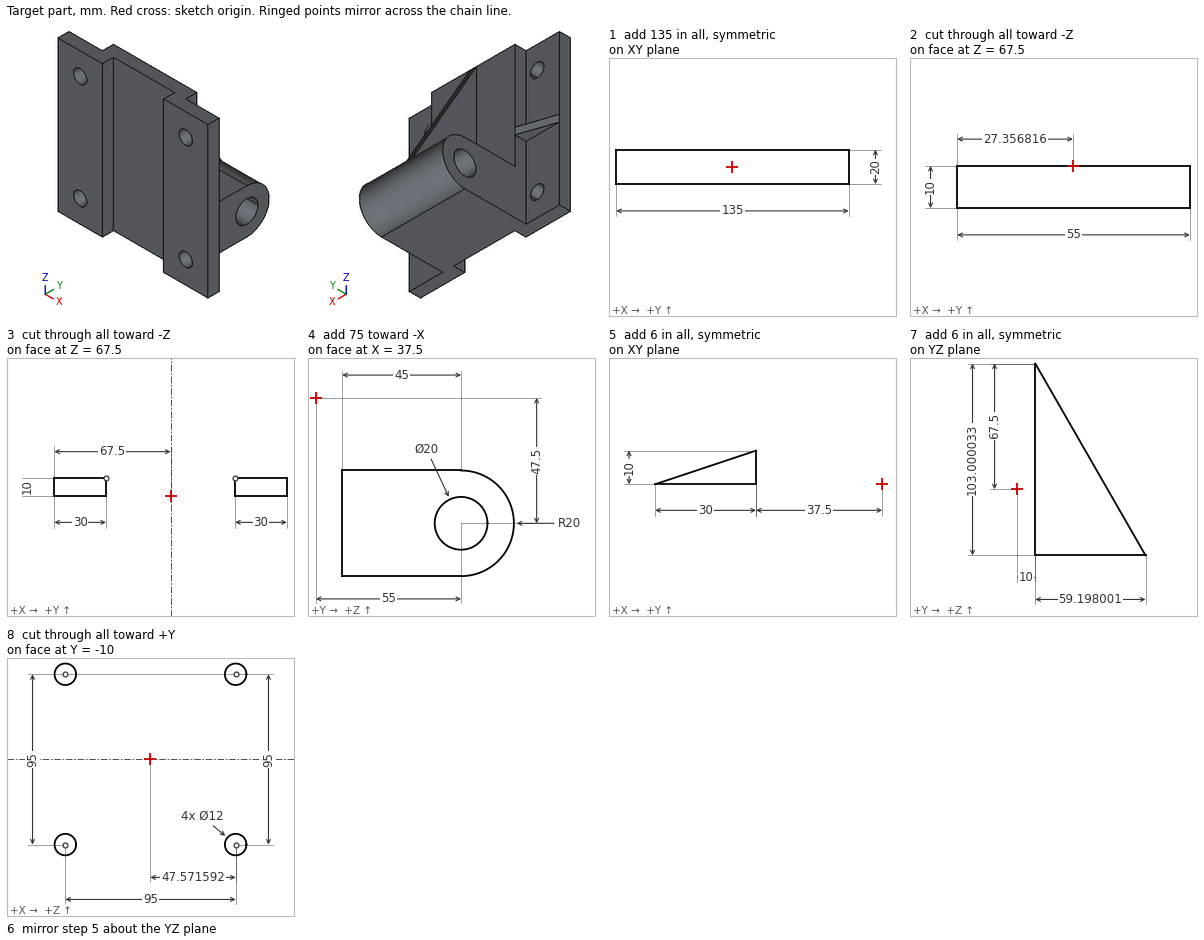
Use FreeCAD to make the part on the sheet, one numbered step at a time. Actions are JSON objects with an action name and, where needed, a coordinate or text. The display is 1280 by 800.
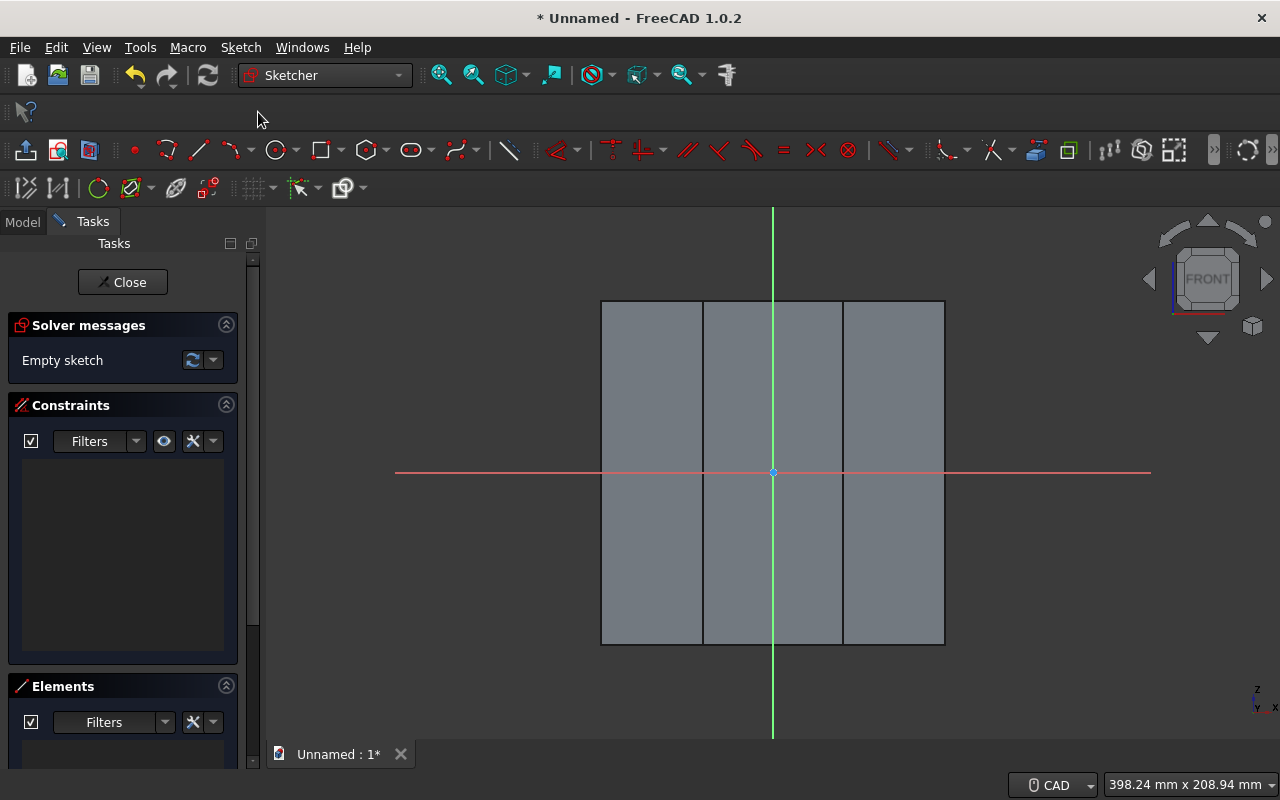
{"action": "left_click", "coordinate": [276, 150]}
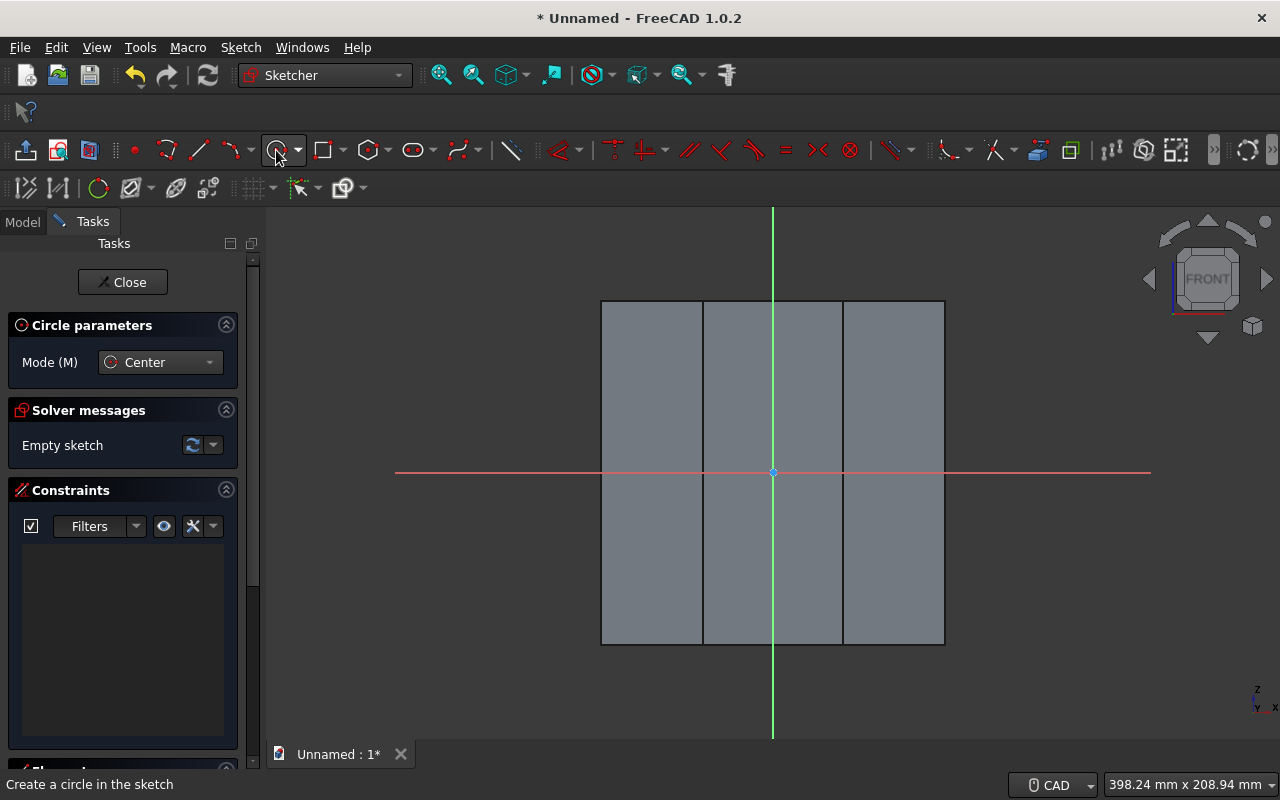
{"action": "scroll", "coordinate": [894, 594], "scroll_direction": "up", "scroll_amount": 2}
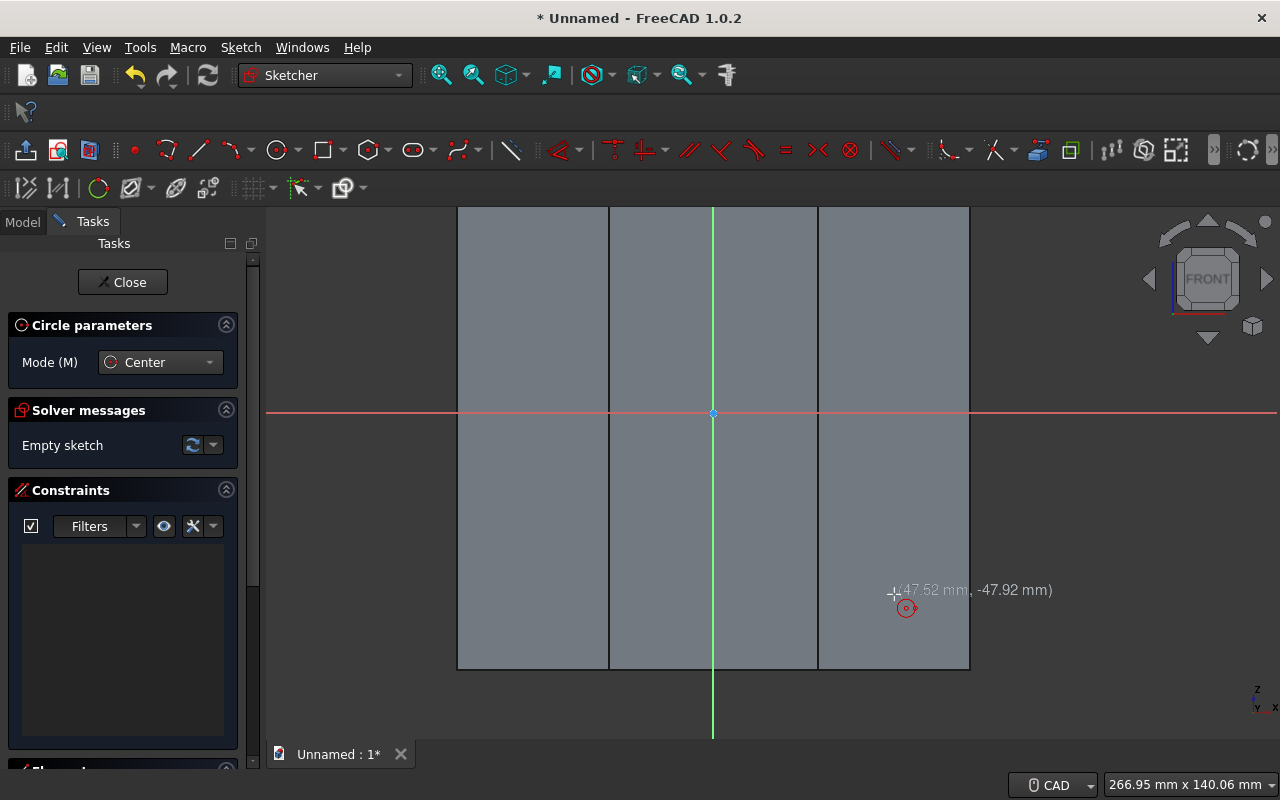
{"action": "left_click", "coordinate": [894, 594]}
{"action": "left_click", "coordinate": [910, 577]}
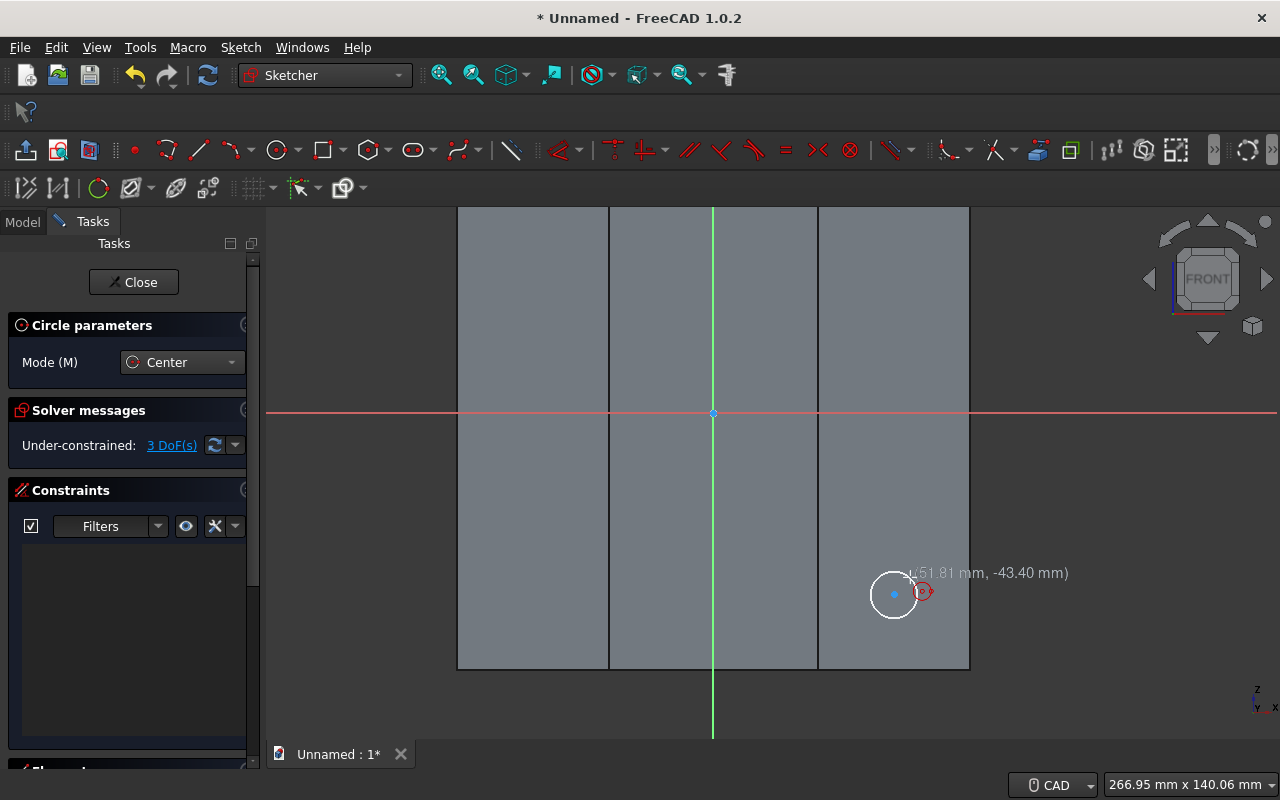
{"action": "left_click", "coordinate": [533, 594]}
{"action": "left_click", "coordinate": [549, 577]}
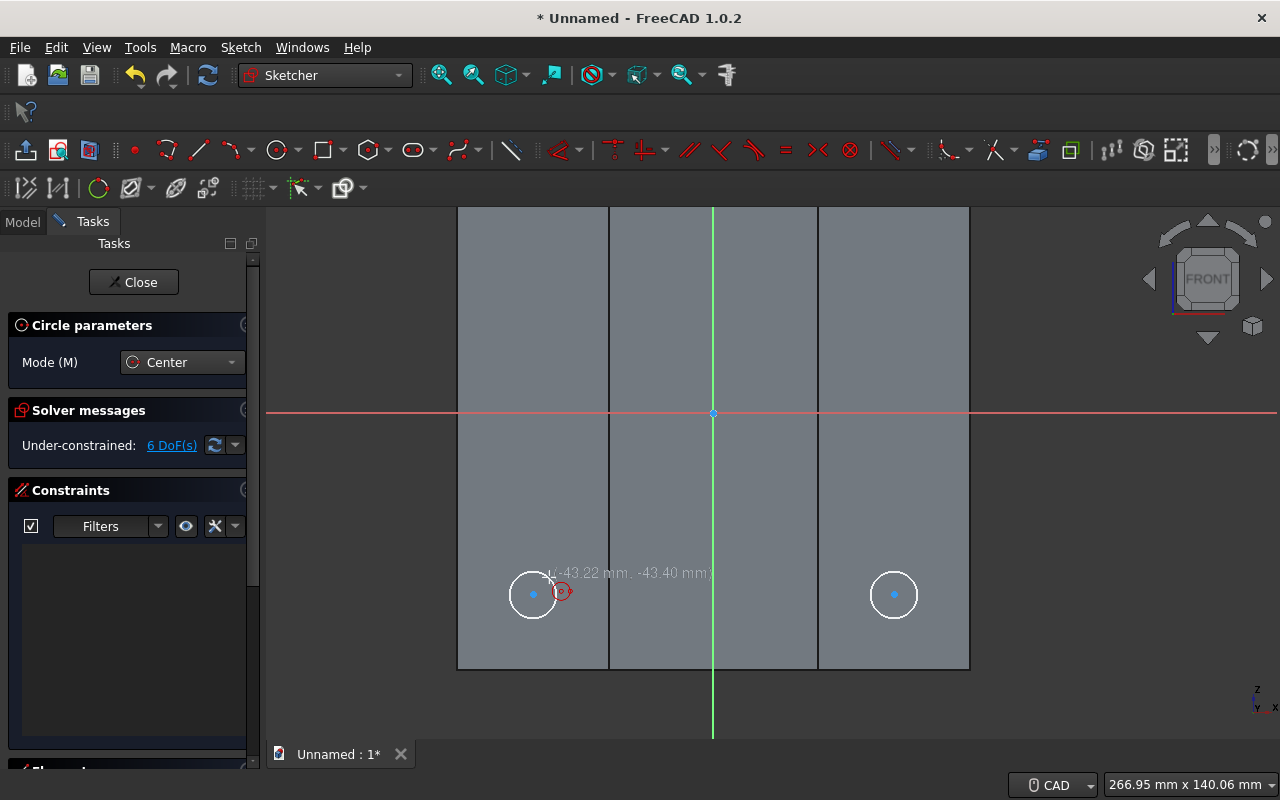
{"action": "scroll", "coordinate": [664, 711], "scroll_direction": "down", "scroll_amount": 1}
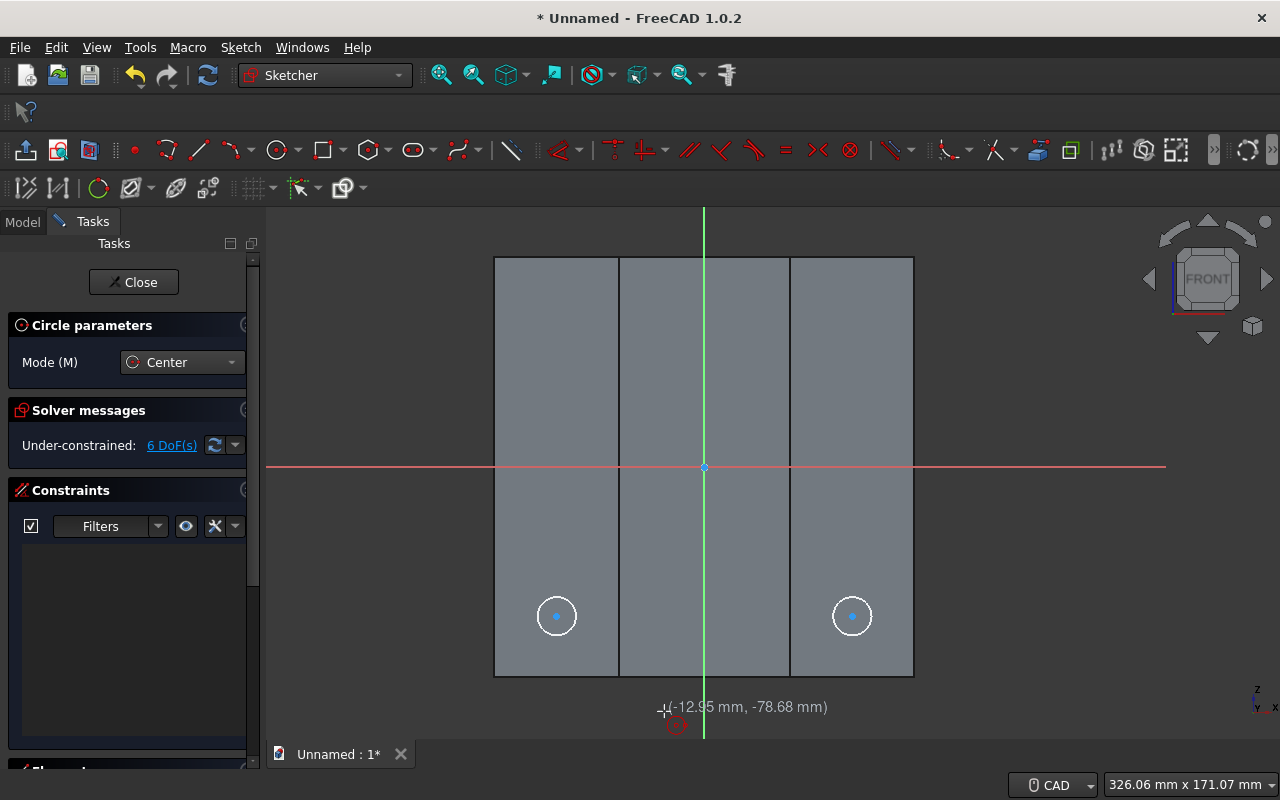
{"action": "left_click", "coordinate": [557, 320]}
{"action": "left_click", "coordinate": [570, 306]}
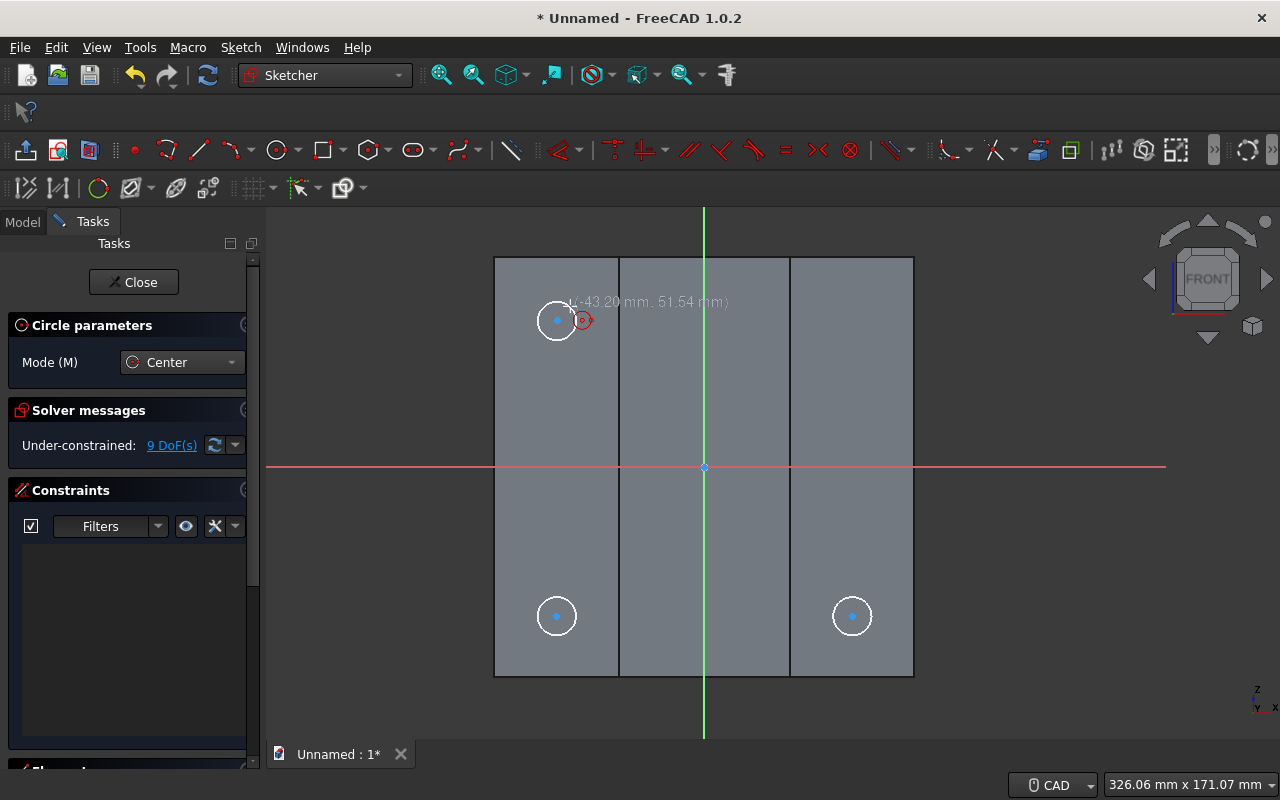
{"action": "left_click", "coordinate": [852, 320]}
{"action": "left_click", "coordinate": [865, 306]}
{"action": "key", "text": "Escape"}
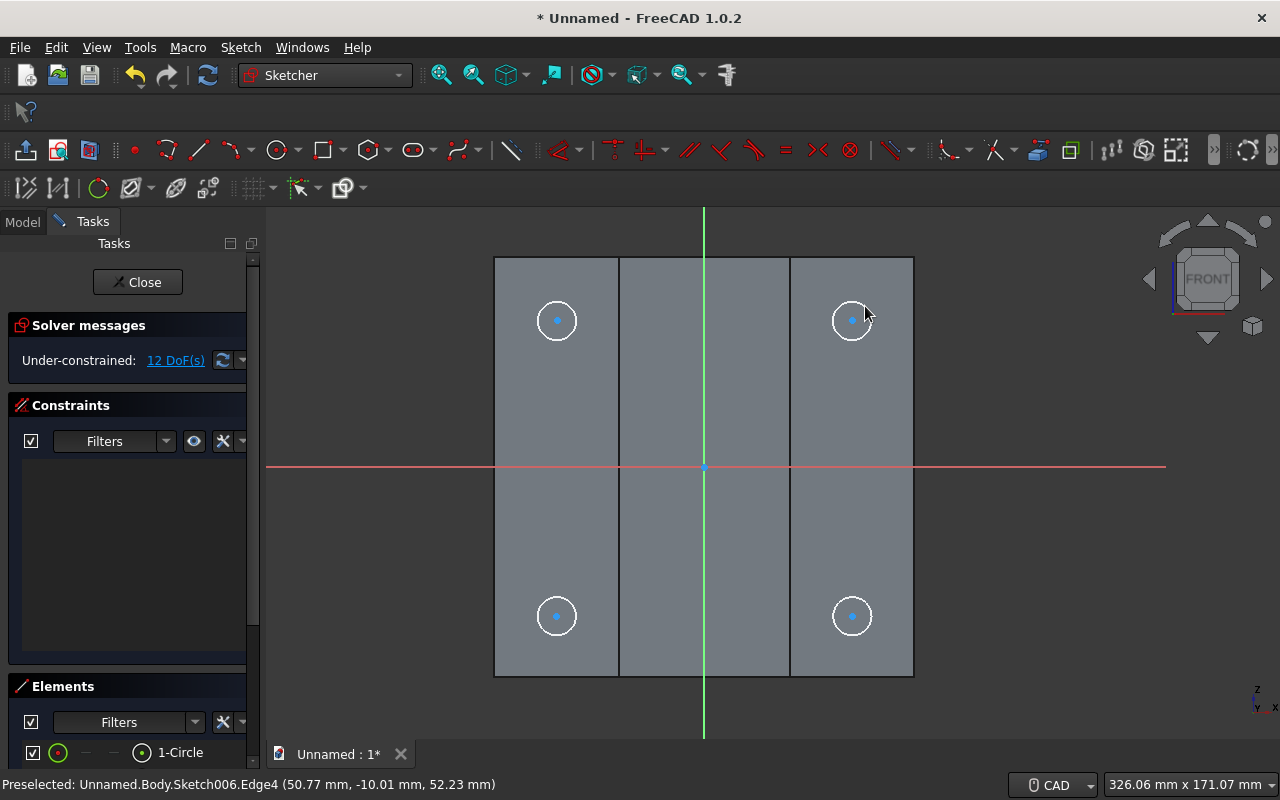
{"action": "left_click", "coordinate": [866, 603]}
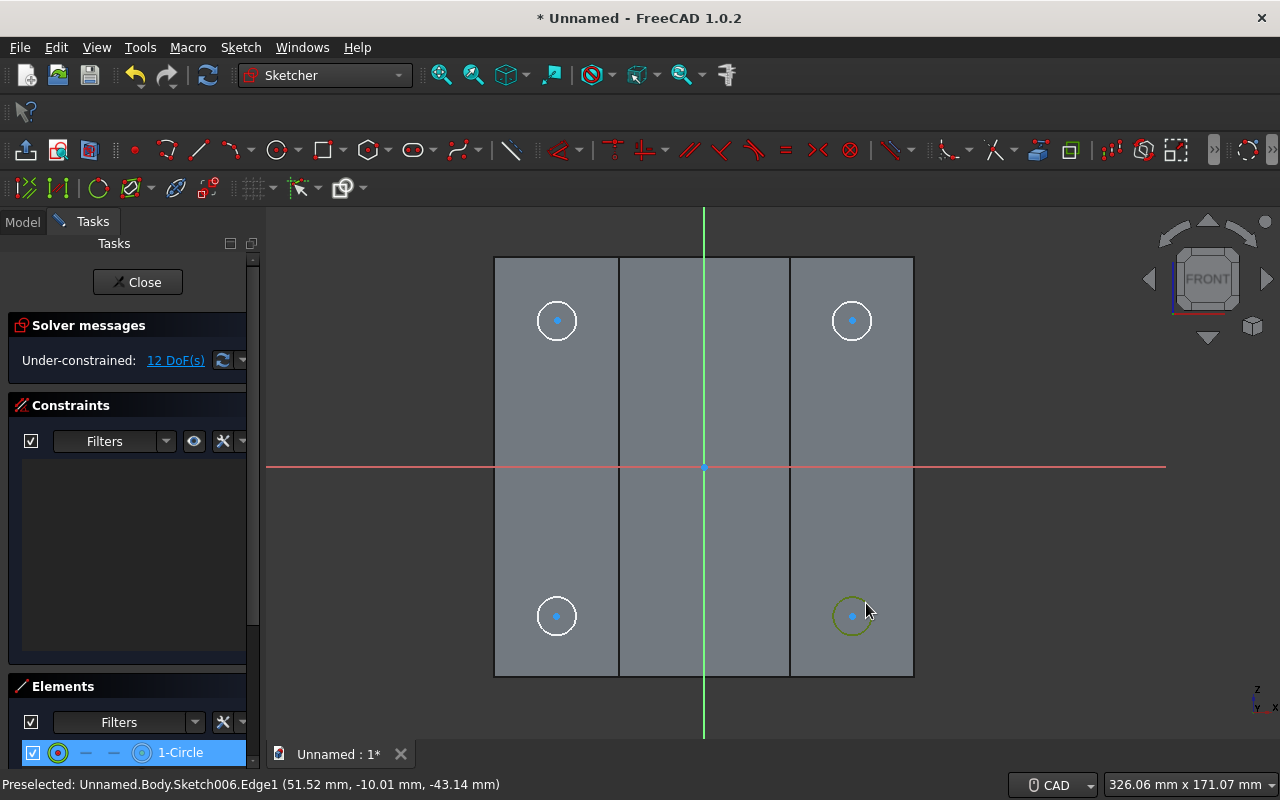
{"action": "left_click", "coordinate": [570, 603]}